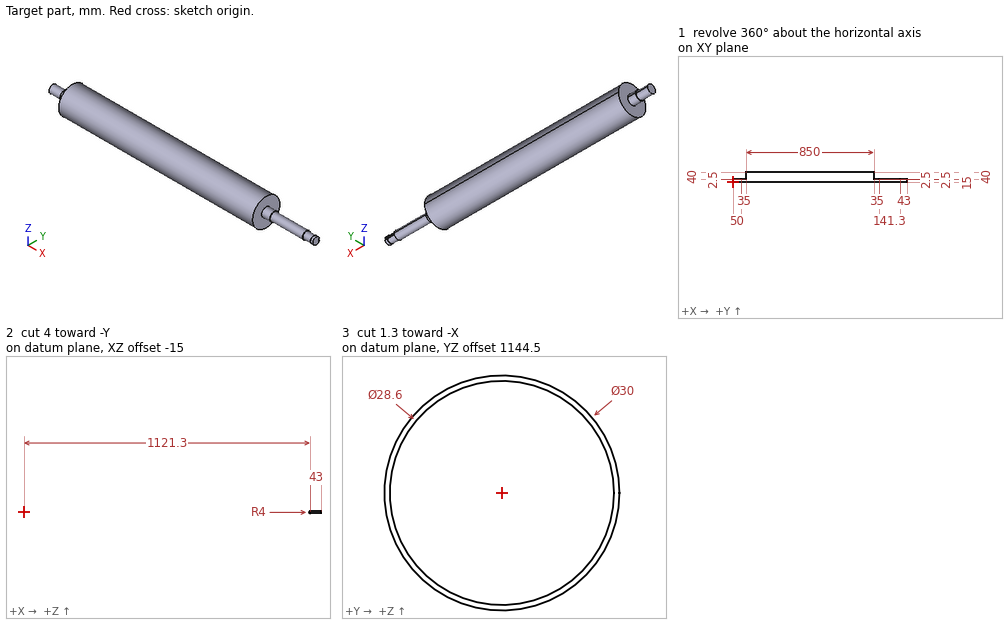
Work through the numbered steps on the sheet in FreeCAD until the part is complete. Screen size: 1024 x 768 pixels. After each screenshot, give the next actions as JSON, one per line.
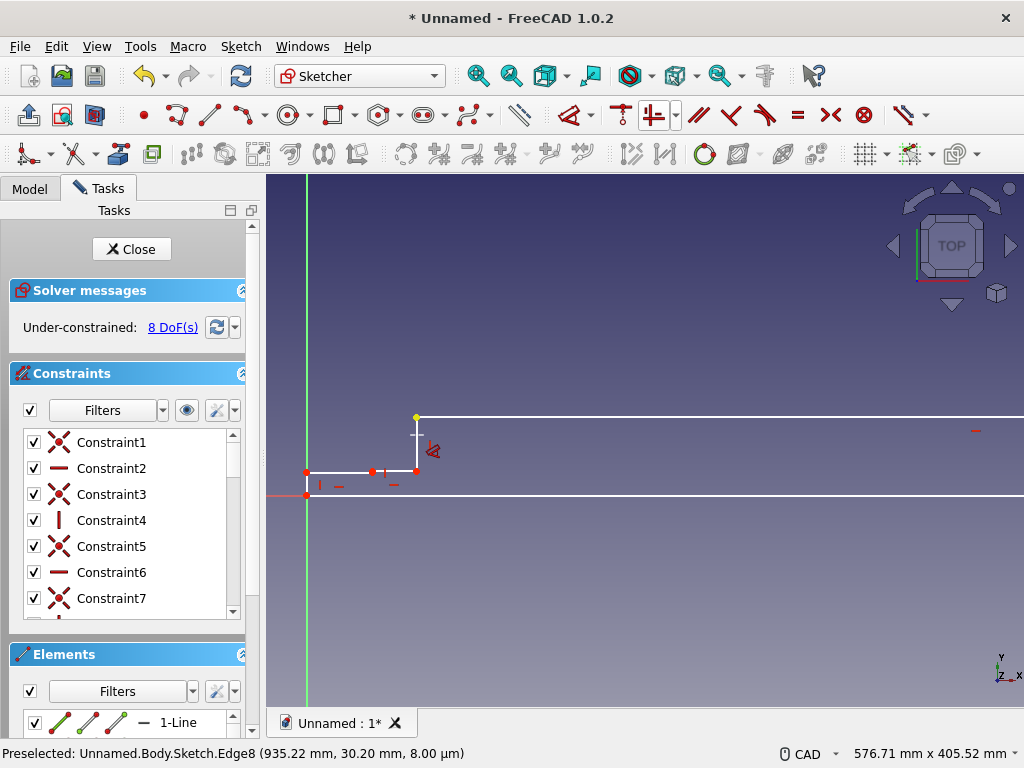
{"action": "left_click", "coordinate": [417, 434]}
{"action": "left_click", "coordinate": [383, 444]}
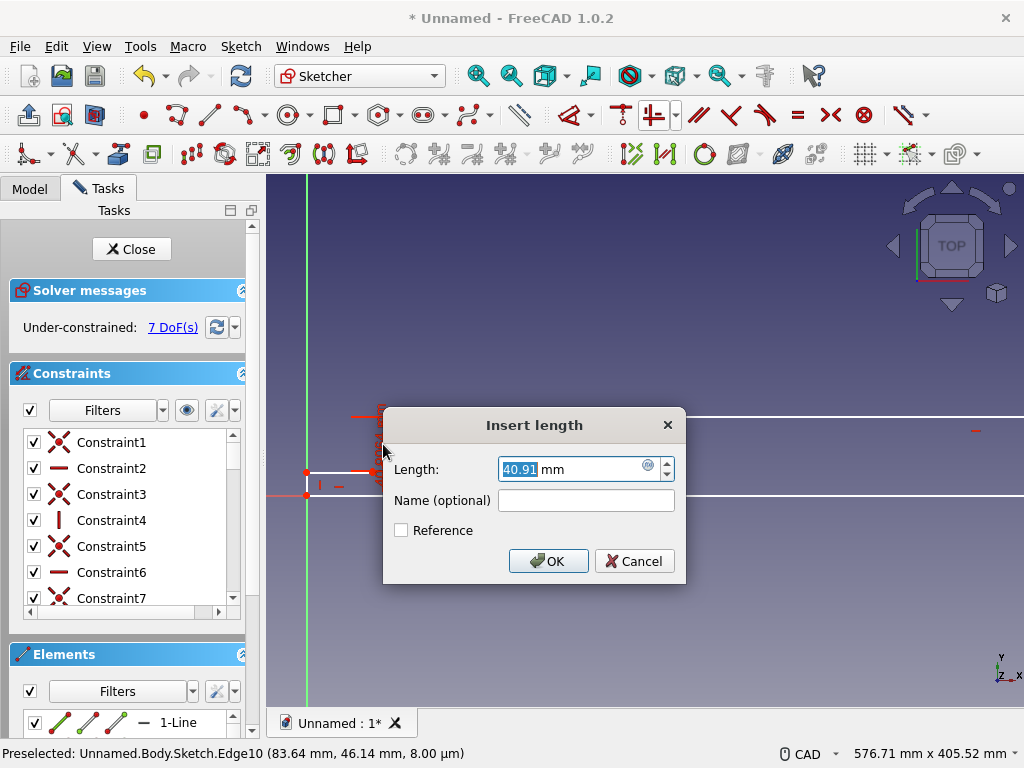
{"action": "type", "text": "40"}
{"action": "key", "text": "Return"}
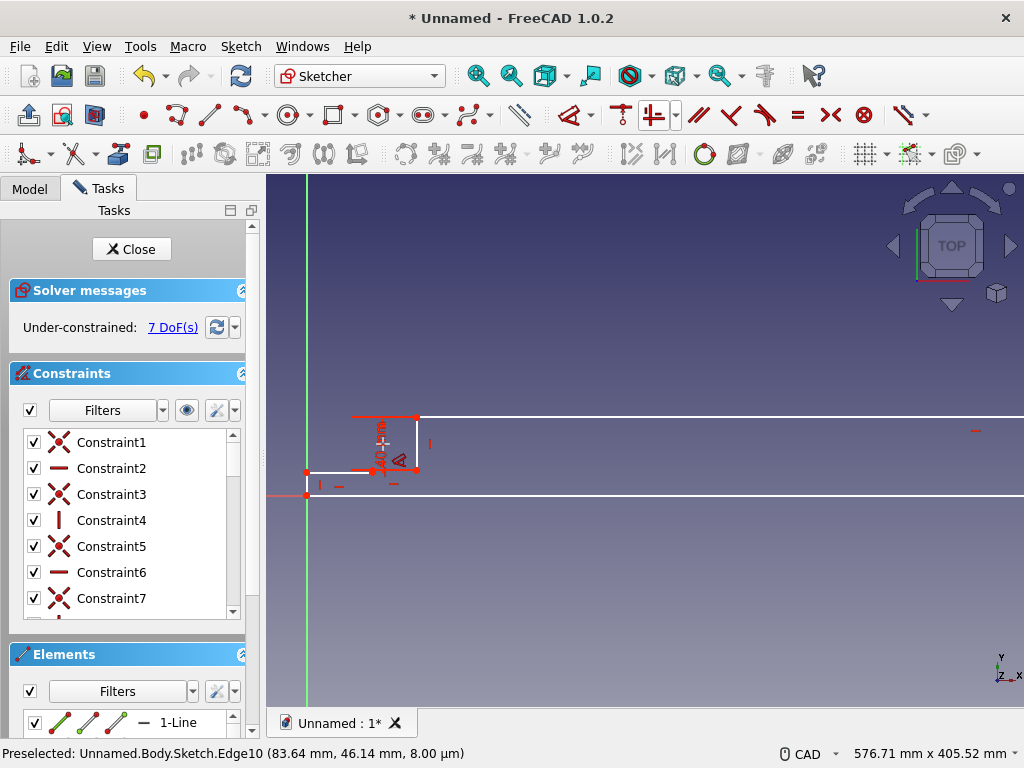
{"action": "left_click", "coordinate": [404, 470]}
{"action": "left_click", "coordinate": [395, 528]}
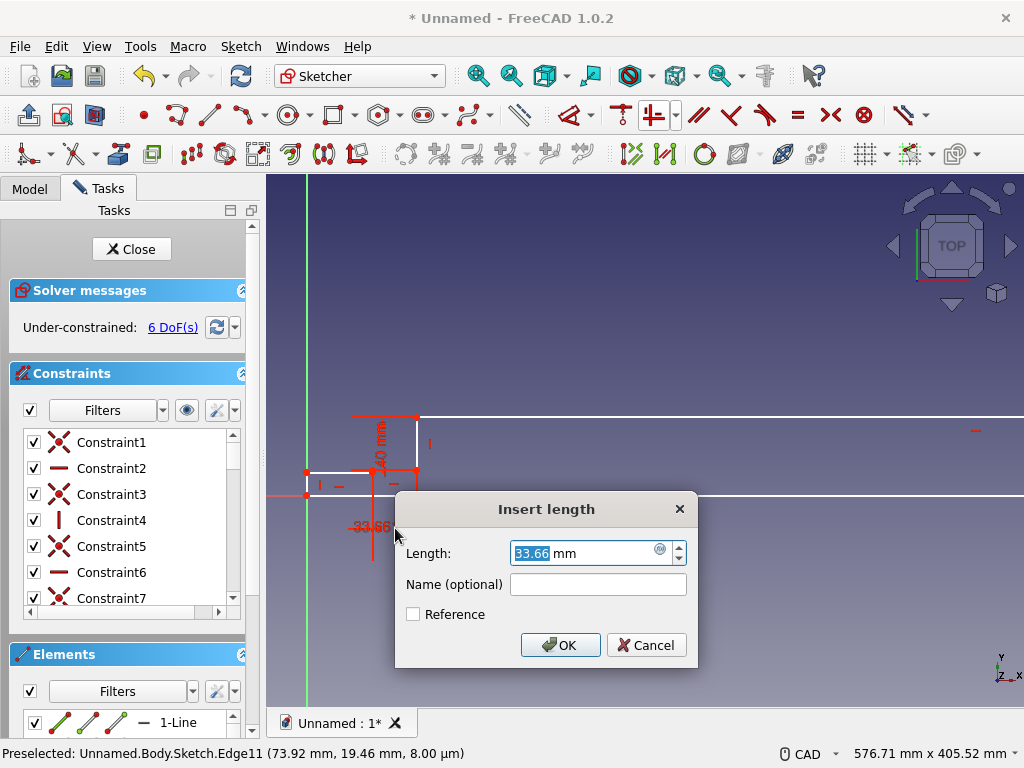
{"action": "type", "text": "35"}
{"action": "key", "text": "Return"}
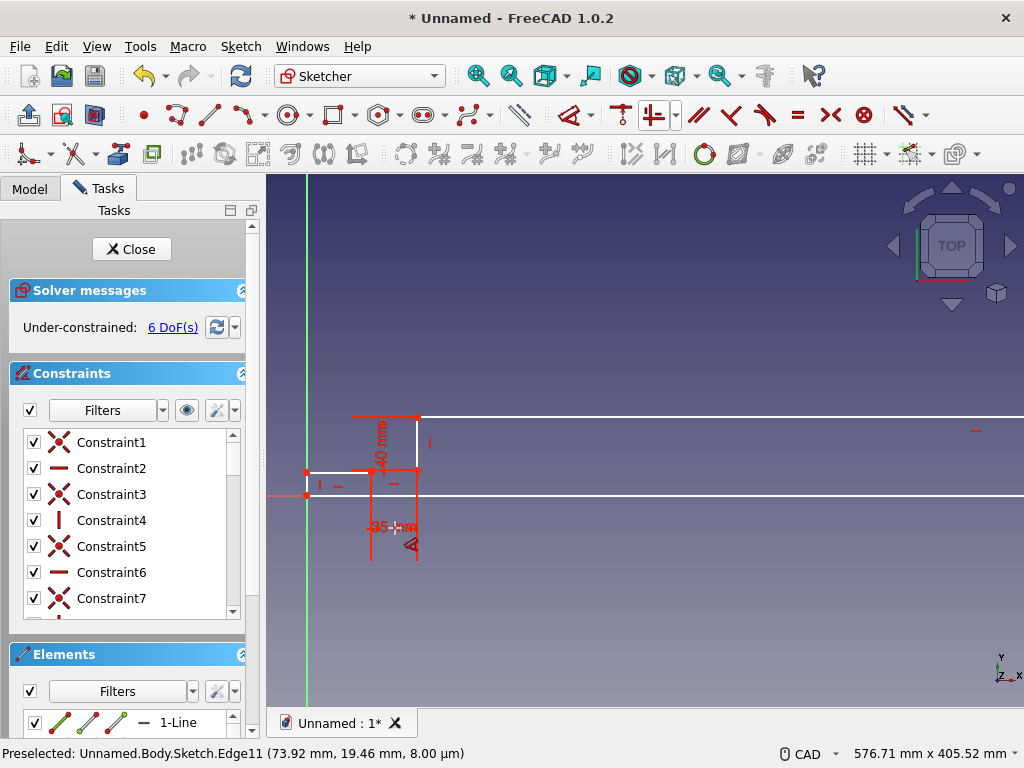
{"action": "left_click", "coordinate": [352, 473]}
{"action": "left_click", "coordinate": [324, 531]}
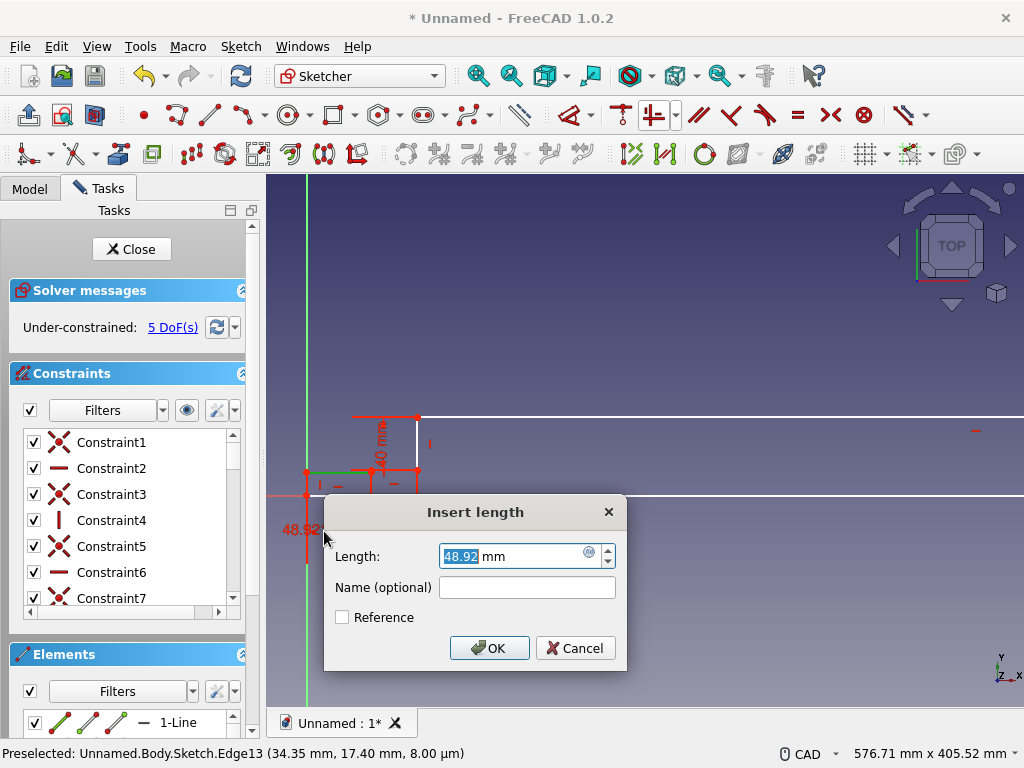
{"action": "type", "text": "50"}
{"action": "key", "text": "Return"}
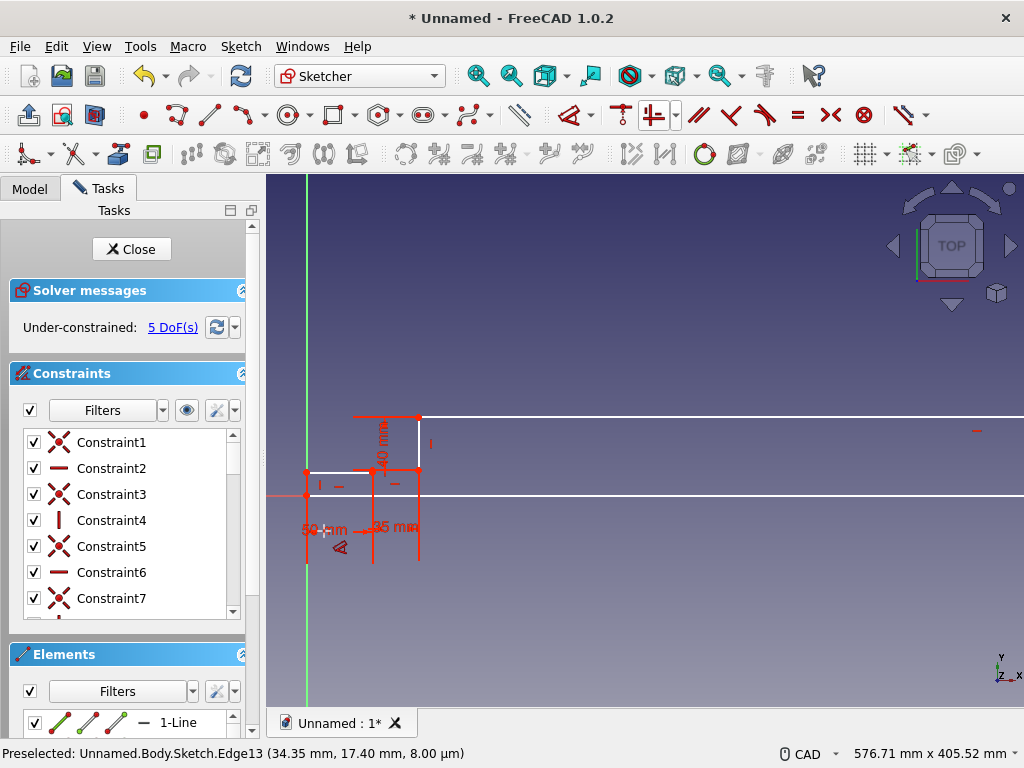
{"action": "scroll", "coordinate": [416, 435], "scroll_direction": "down", "scroll_amount": 7}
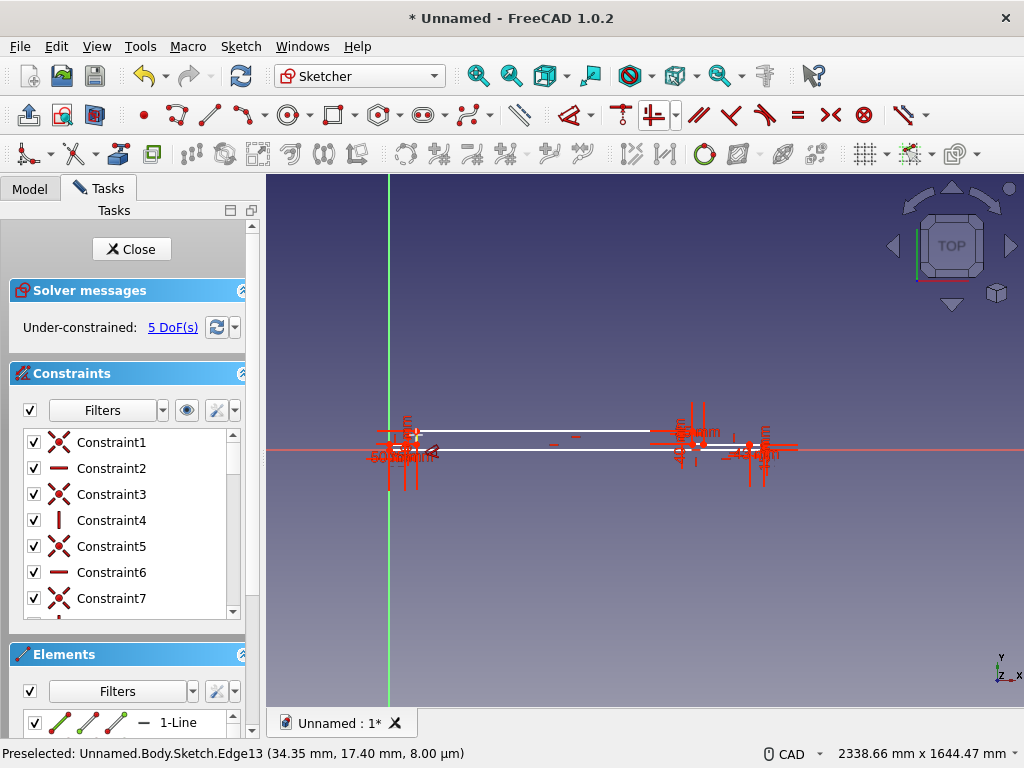
{"action": "scroll", "coordinate": [750, 445], "scroll_direction": "up", "scroll_amount": 20}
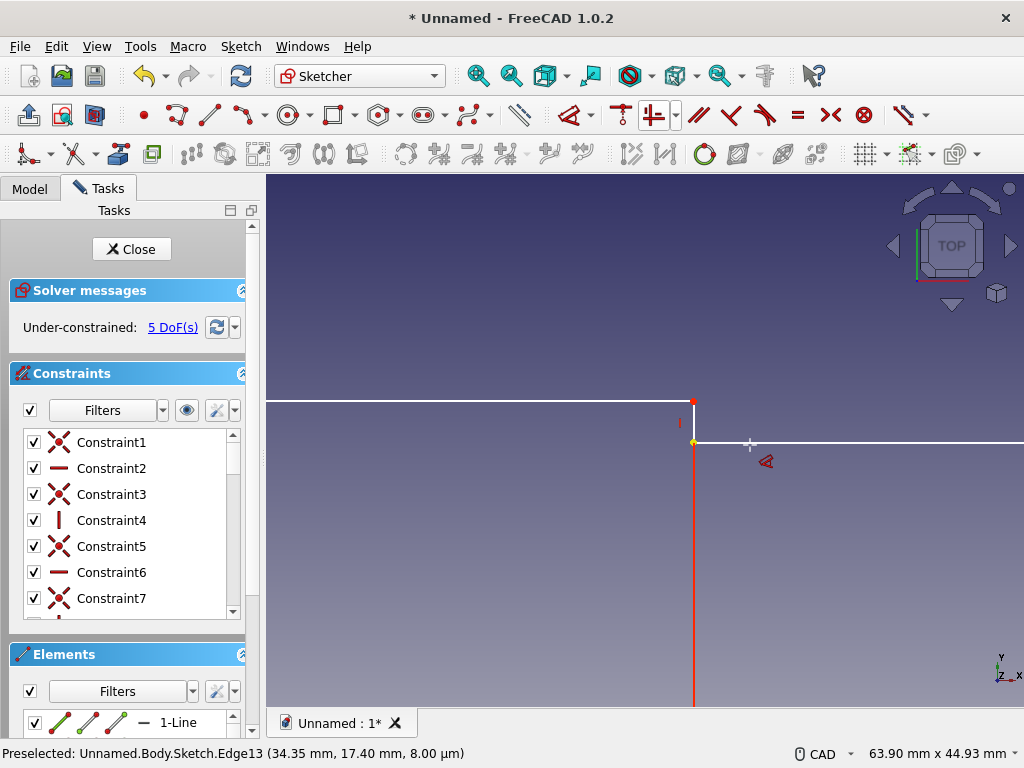
{"action": "left_click", "coordinate": [694, 422]}
{"action": "left_click", "coordinate": [728, 422]}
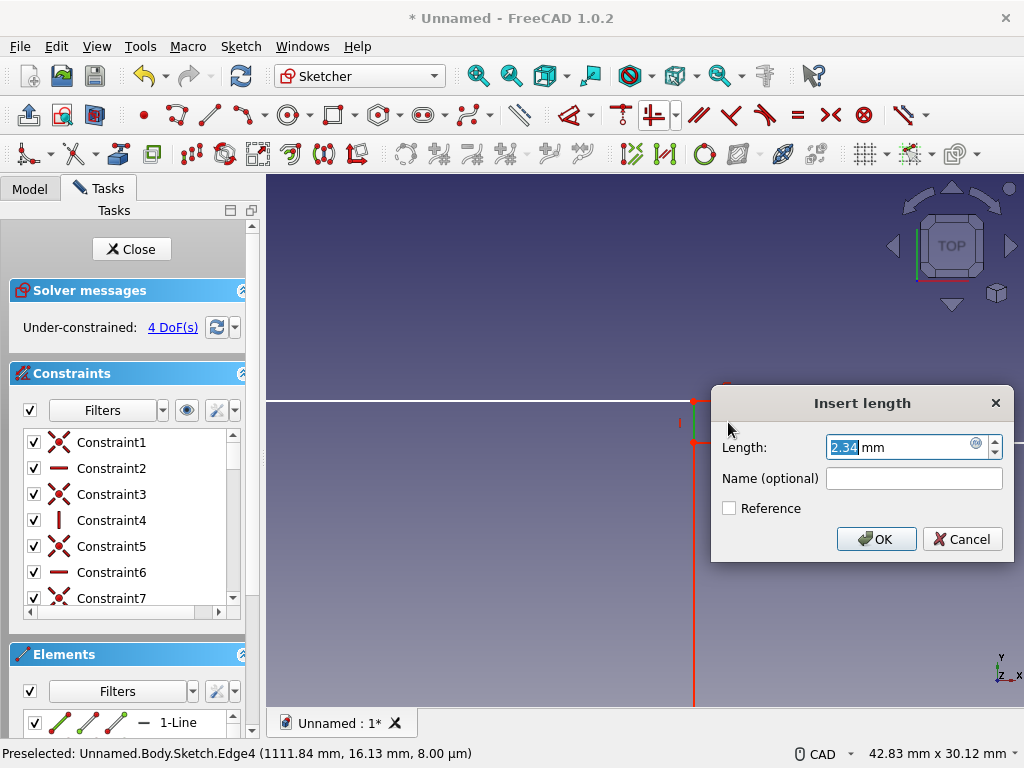
{"action": "type", "text": "2.5"}
{"action": "key", "text": "Return"}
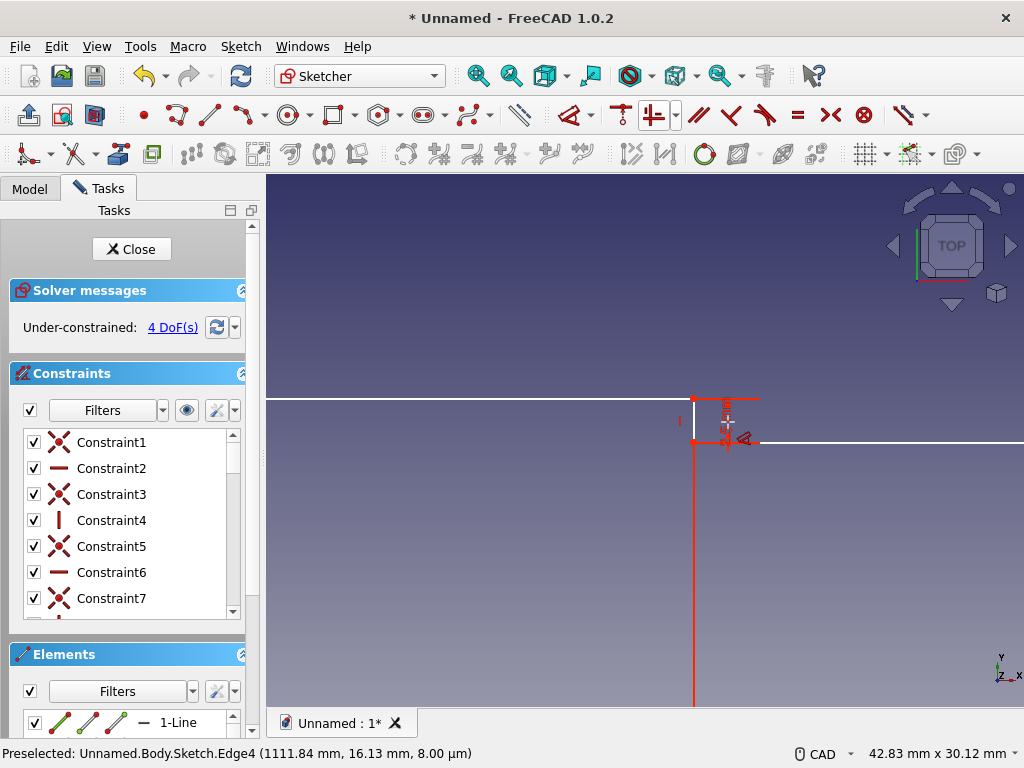
{"action": "scroll", "coordinate": [576, 440], "scroll_direction": "down", "scroll_amount": 15}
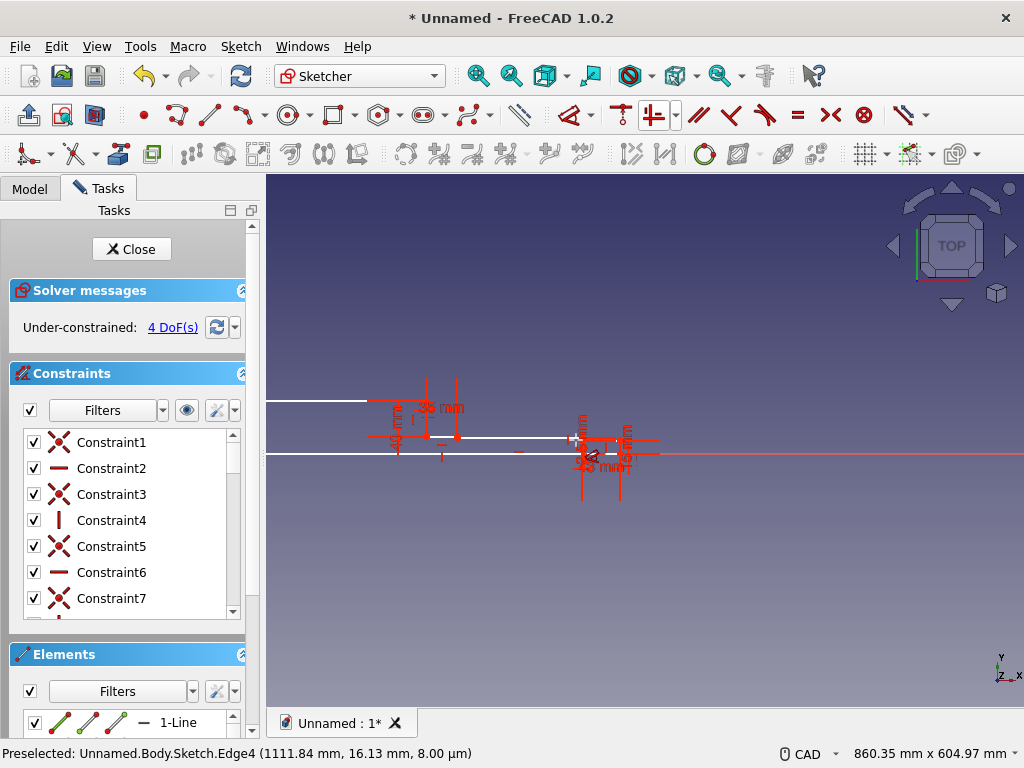
{"action": "scroll", "coordinate": [847, 448], "scroll_direction": "down", "scroll_amount": 5}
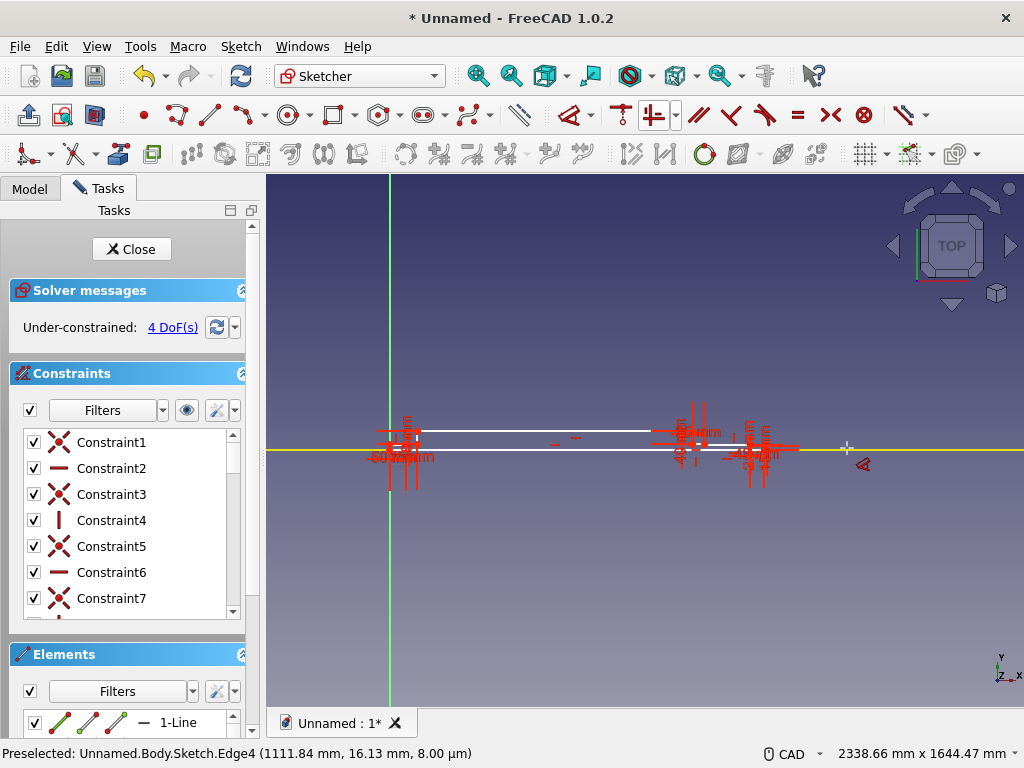
{"action": "scroll", "coordinate": [704, 445], "scroll_direction": "up", "scroll_amount": 20}